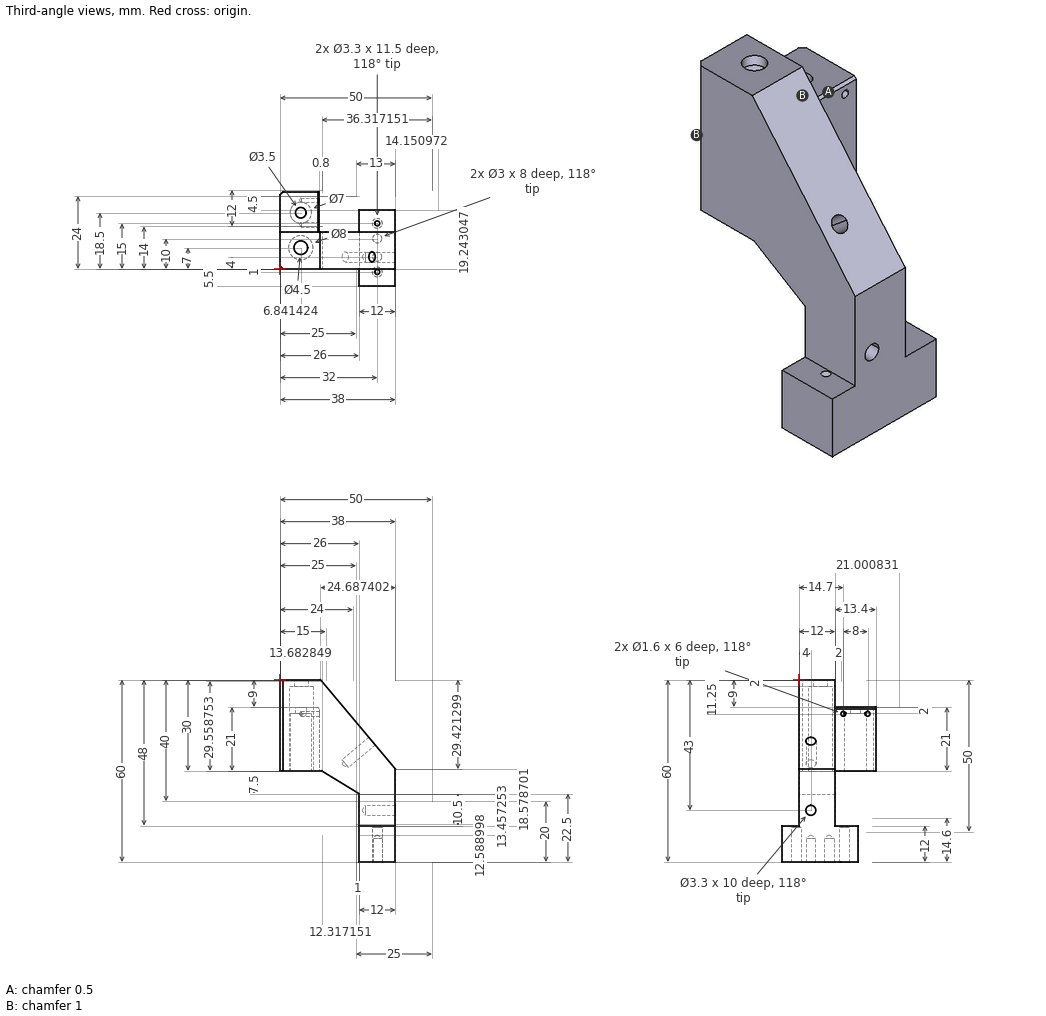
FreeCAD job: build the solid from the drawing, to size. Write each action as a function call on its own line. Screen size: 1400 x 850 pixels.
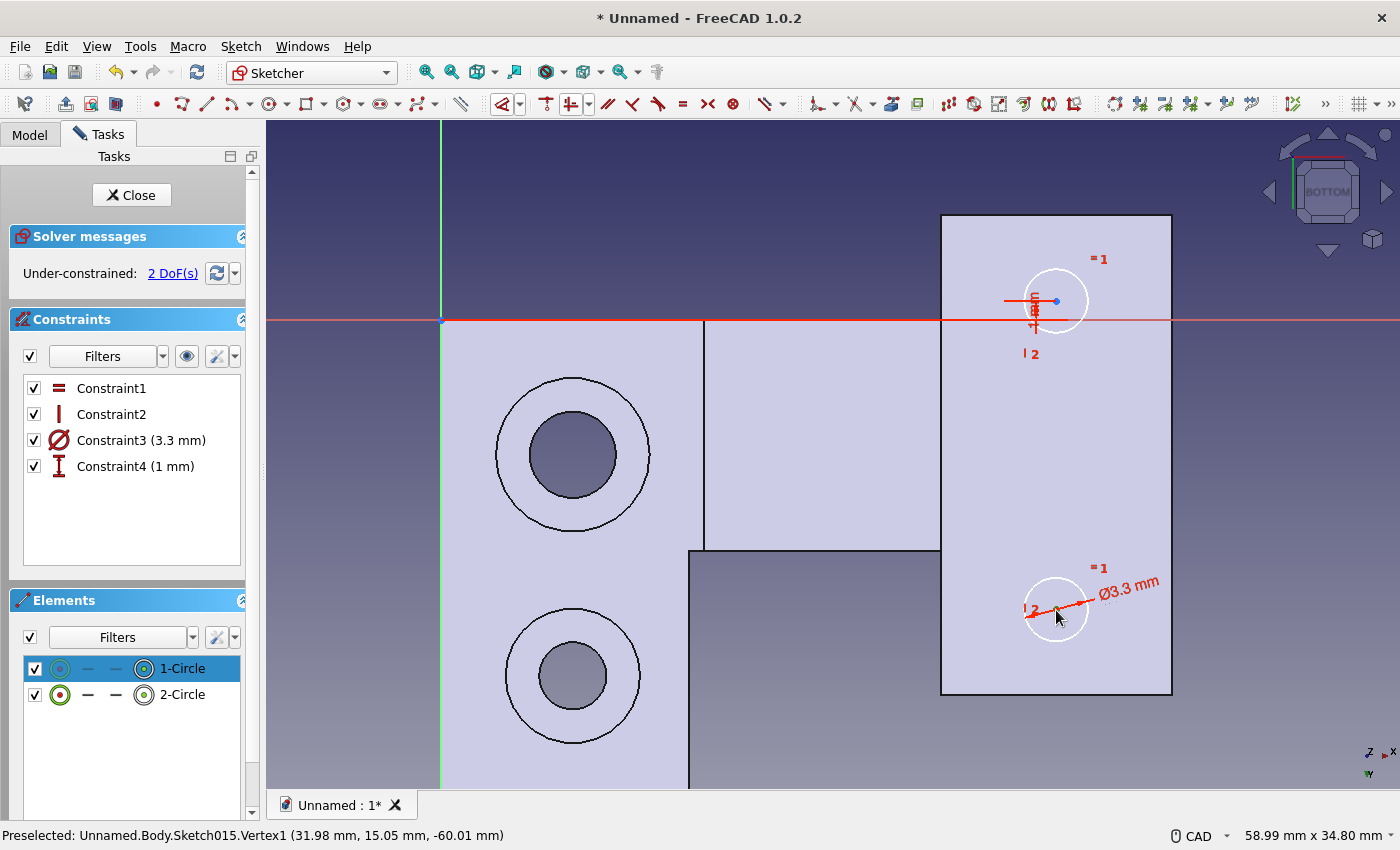
click(520, 104)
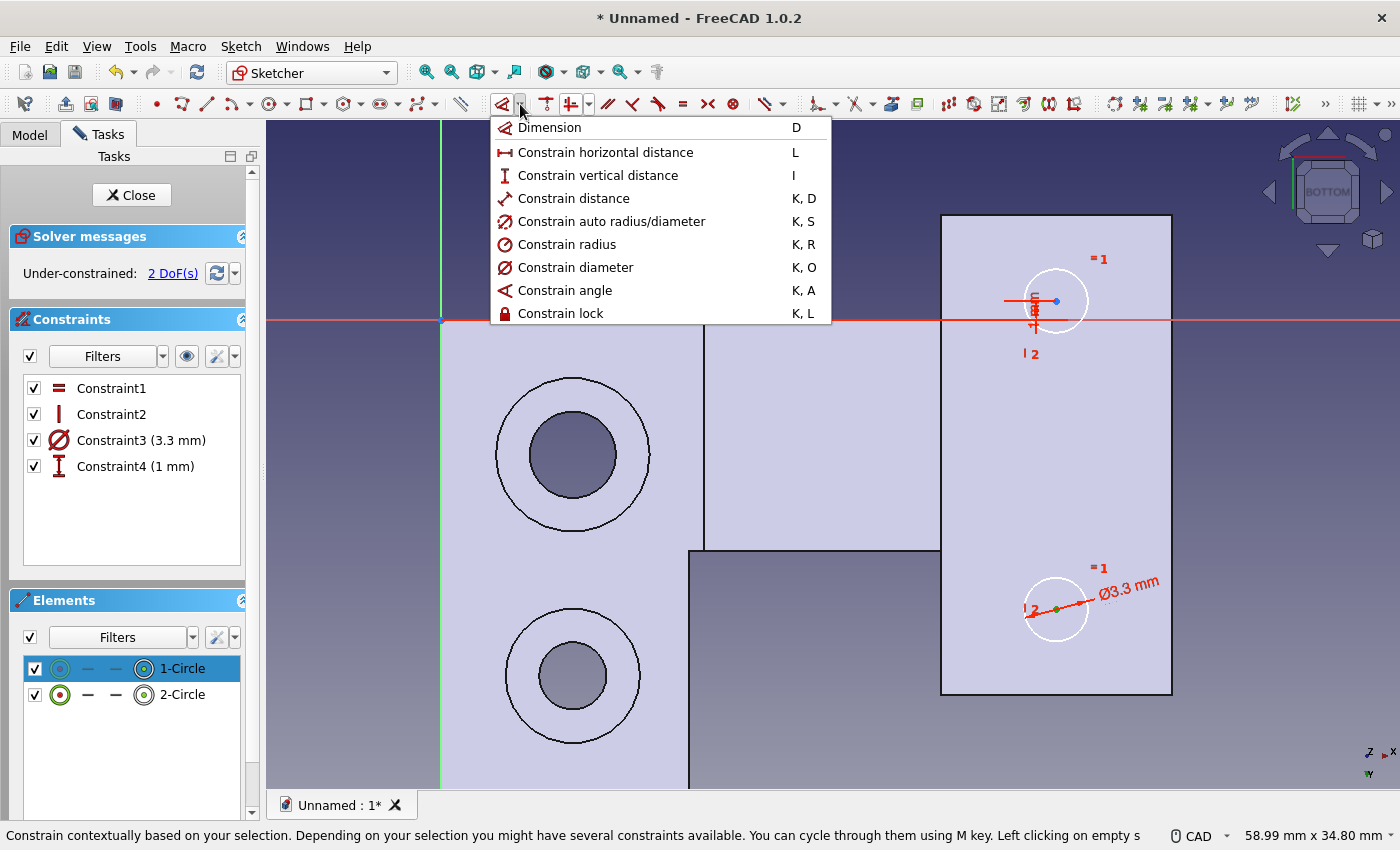
click(661, 152)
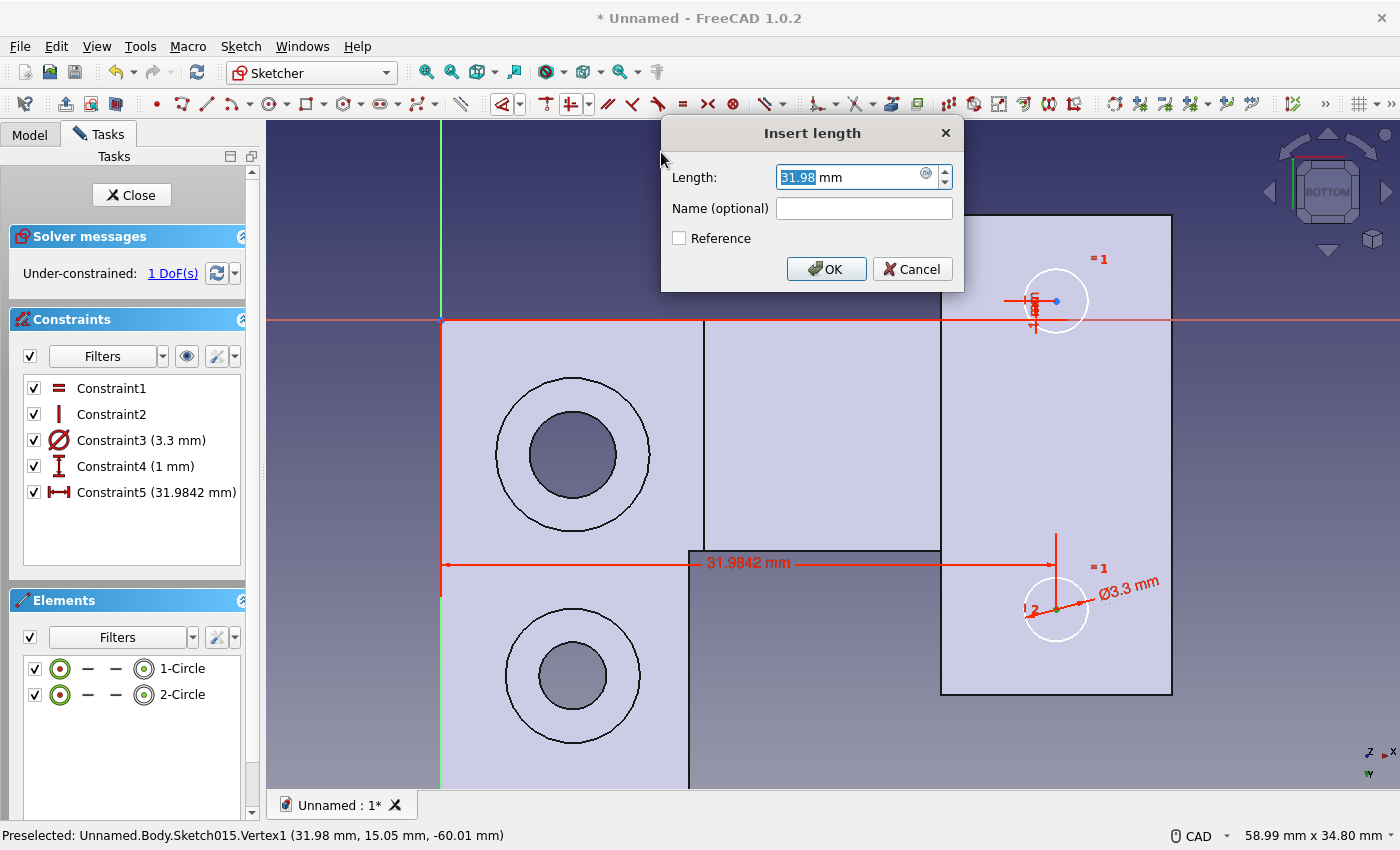
text(32)
key(Return)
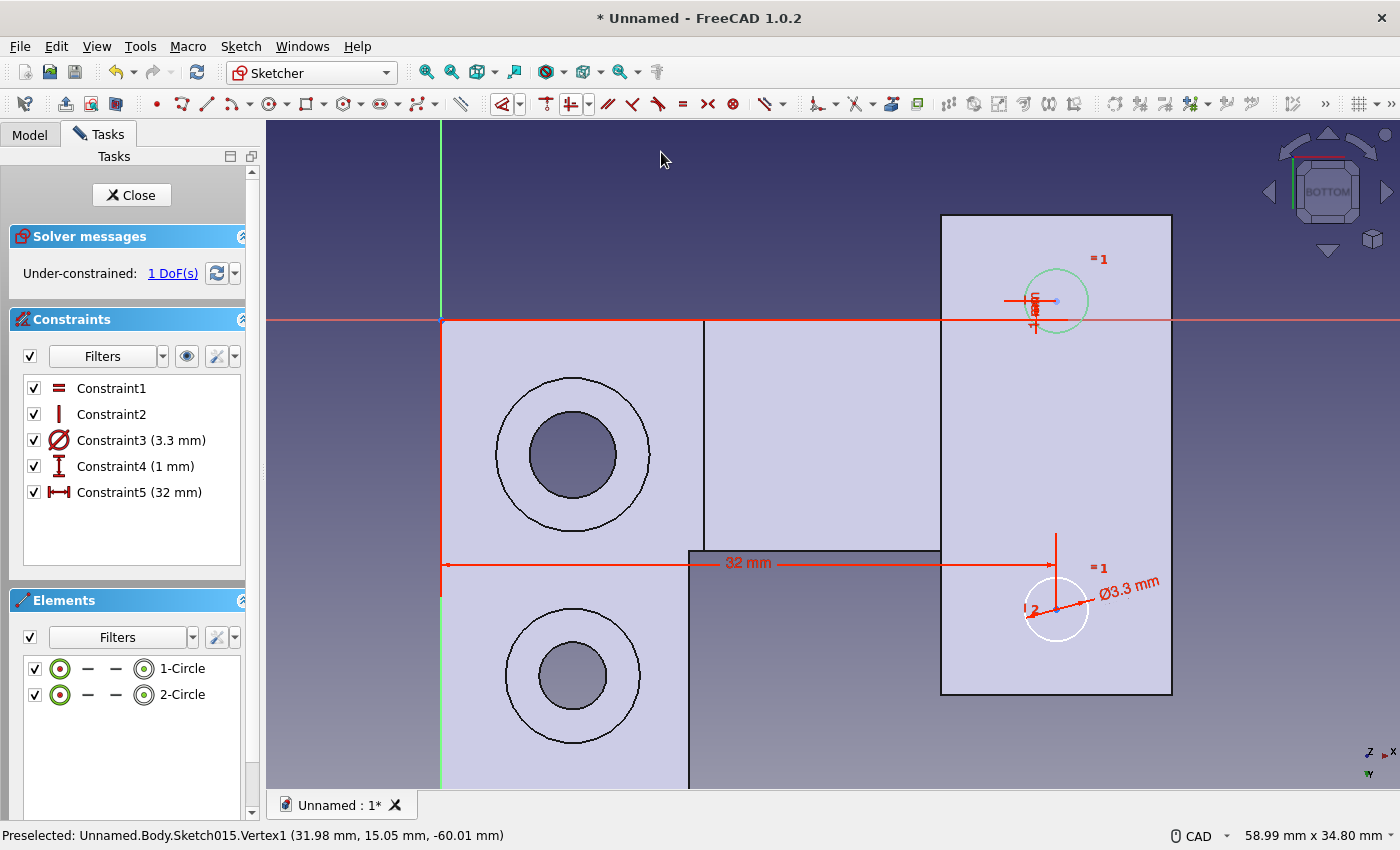
click(1056, 610)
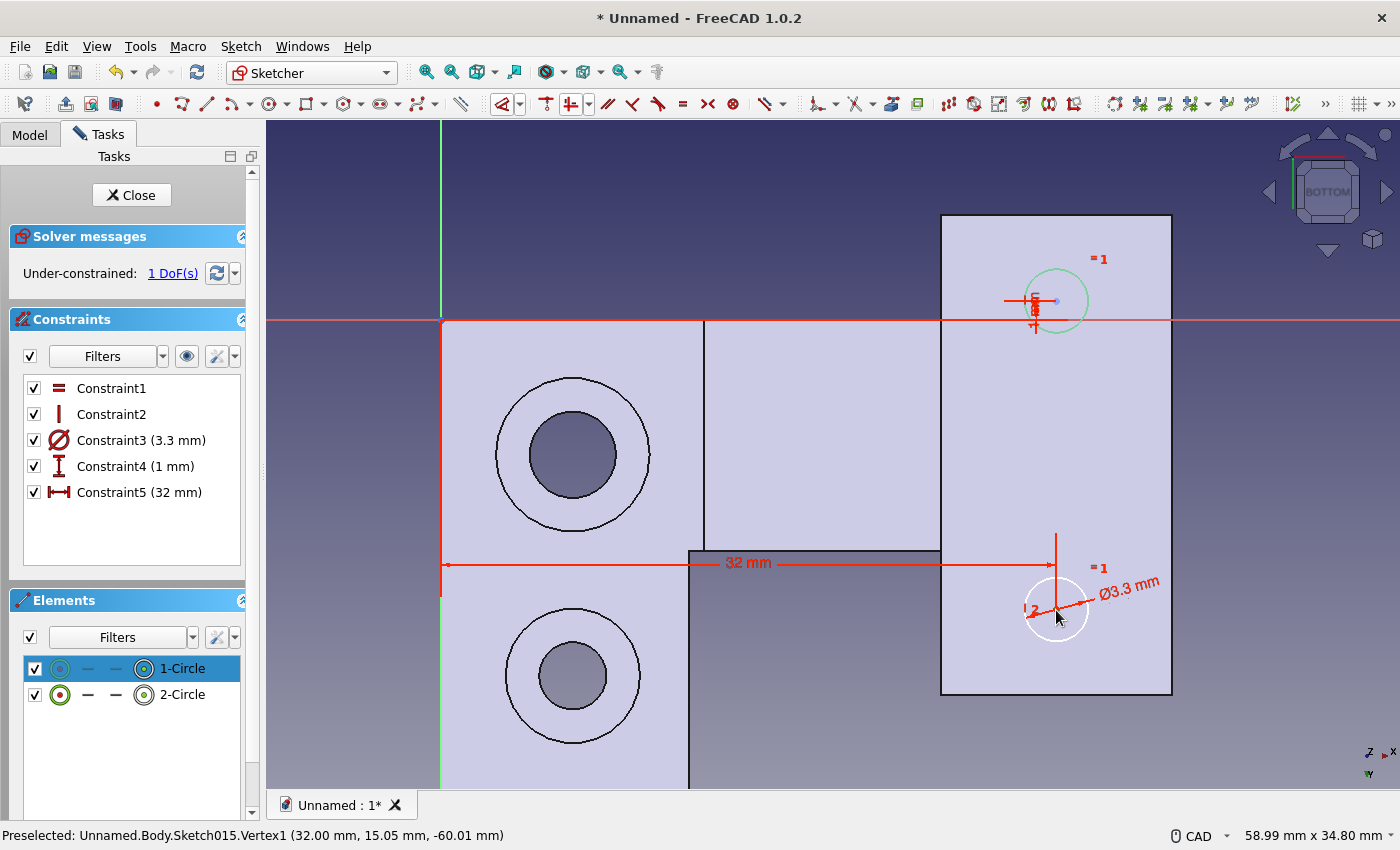
click(520, 104)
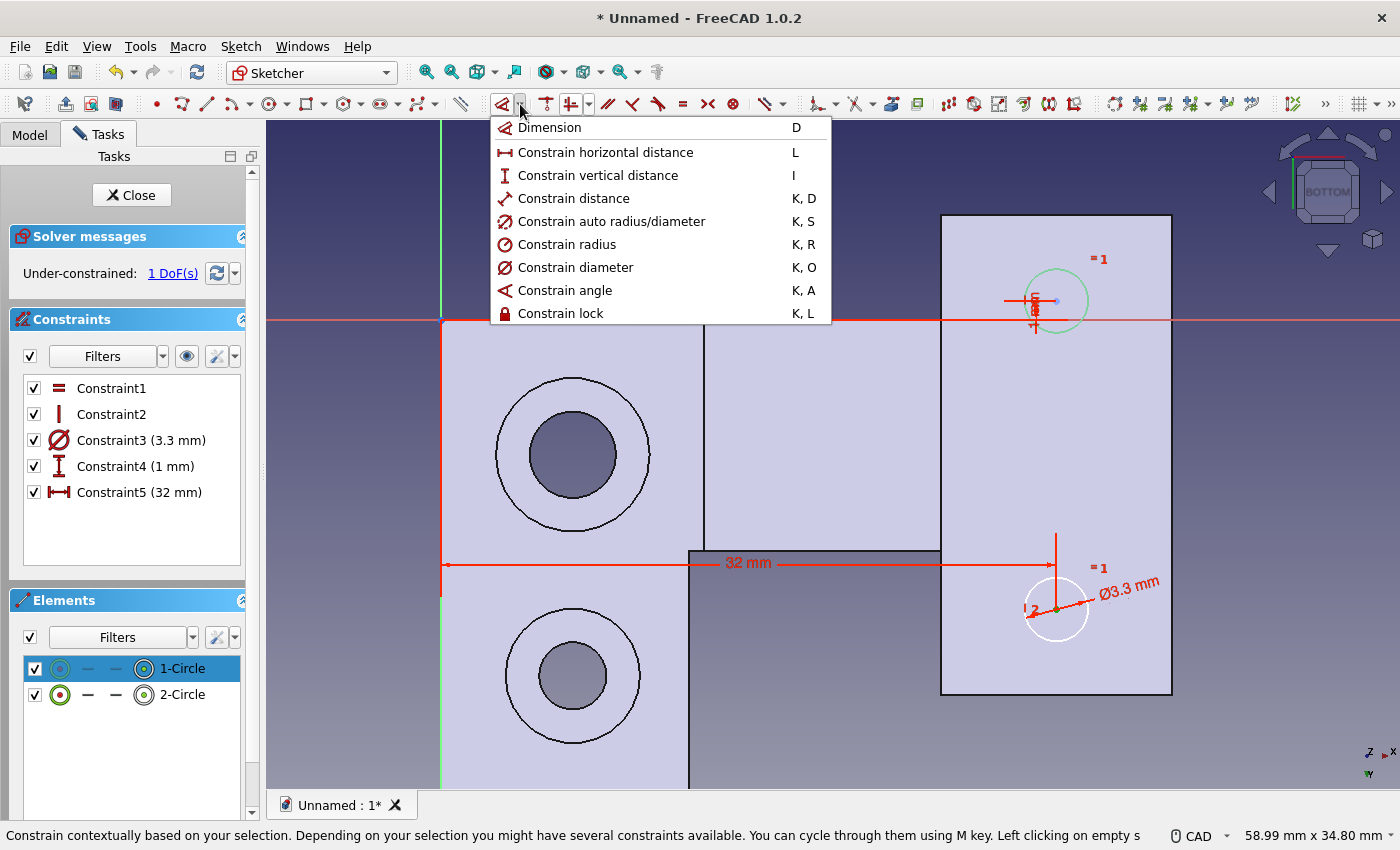
click(661, 176)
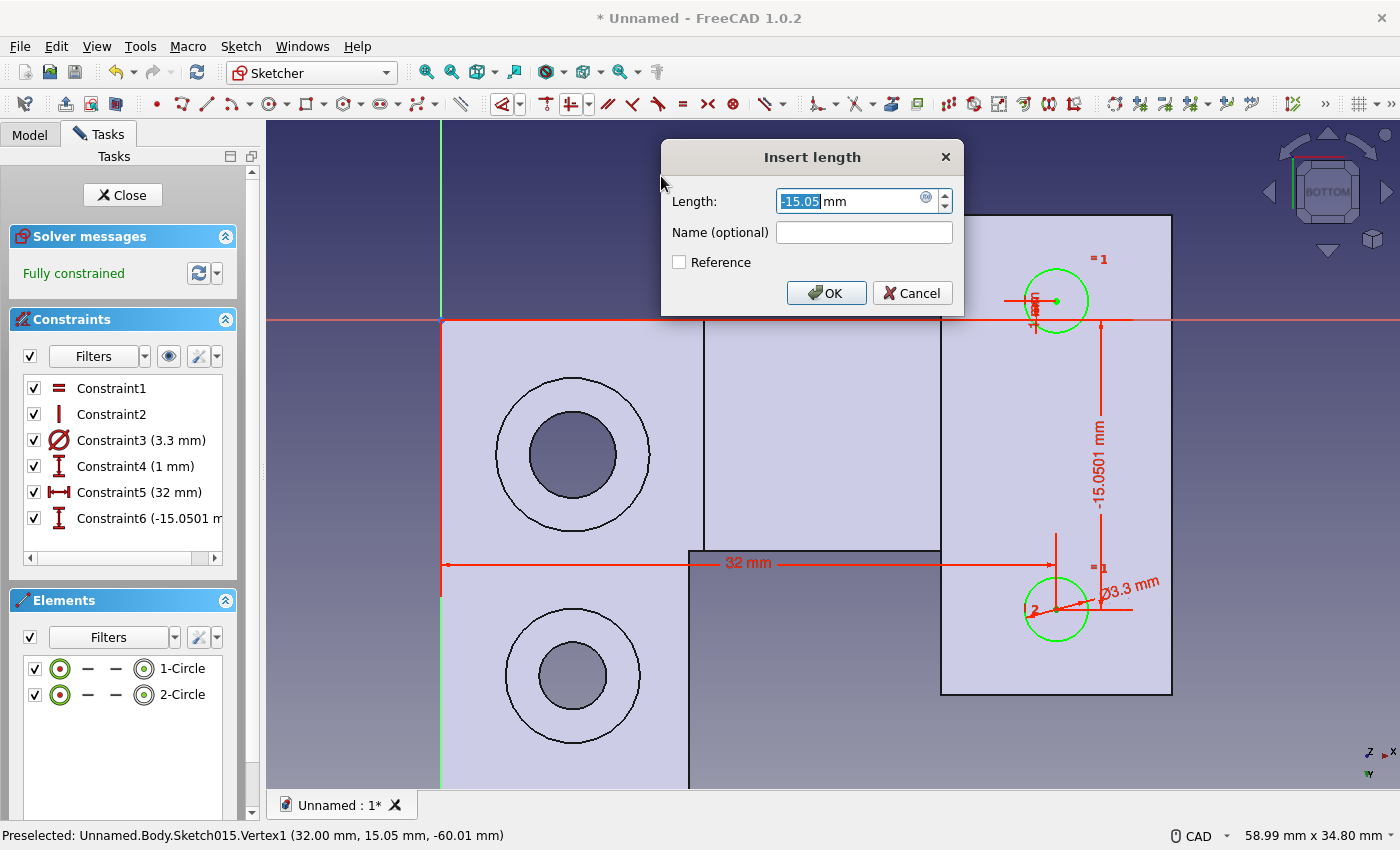
text(-15)
key(Return)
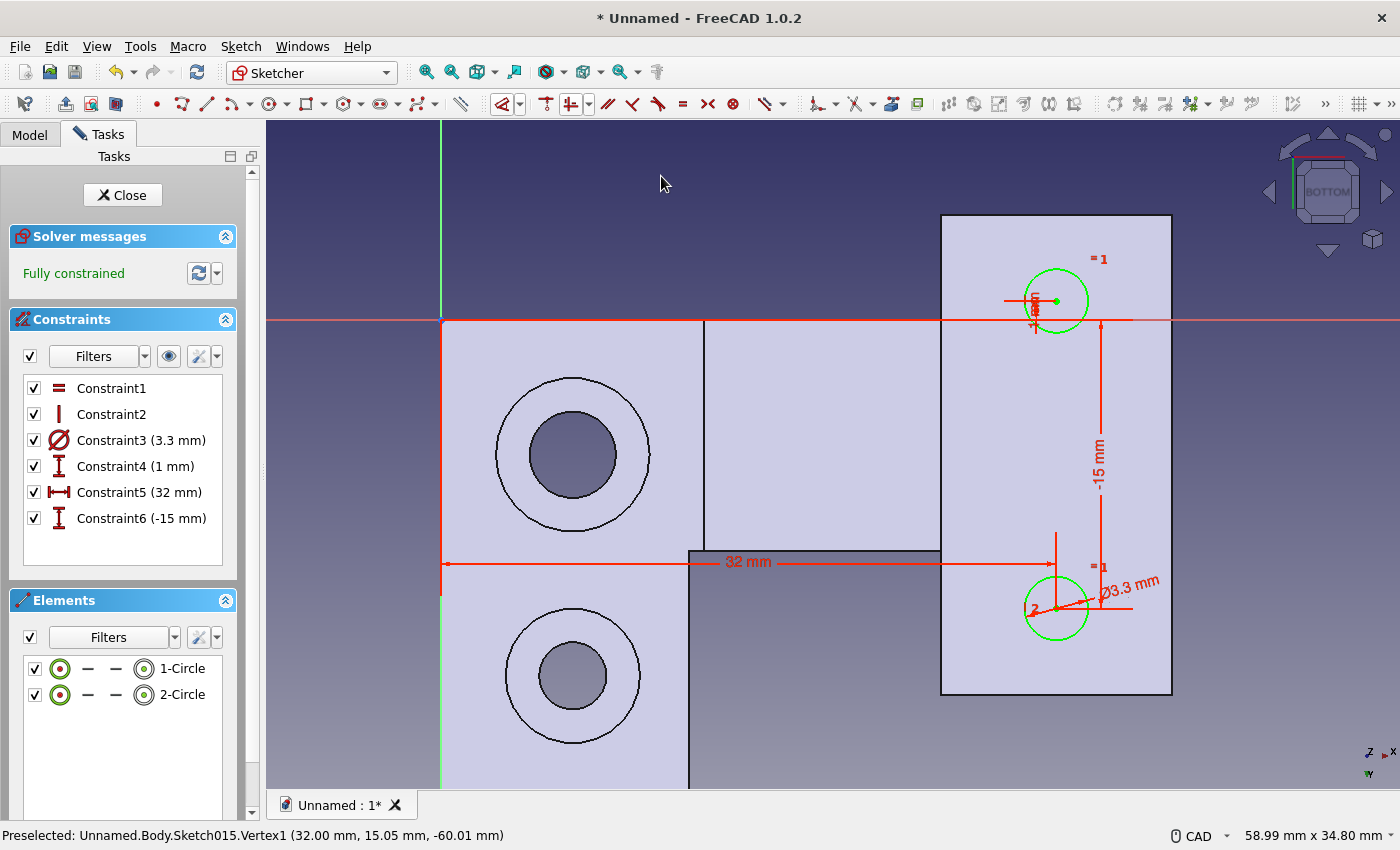
click(123, 195)